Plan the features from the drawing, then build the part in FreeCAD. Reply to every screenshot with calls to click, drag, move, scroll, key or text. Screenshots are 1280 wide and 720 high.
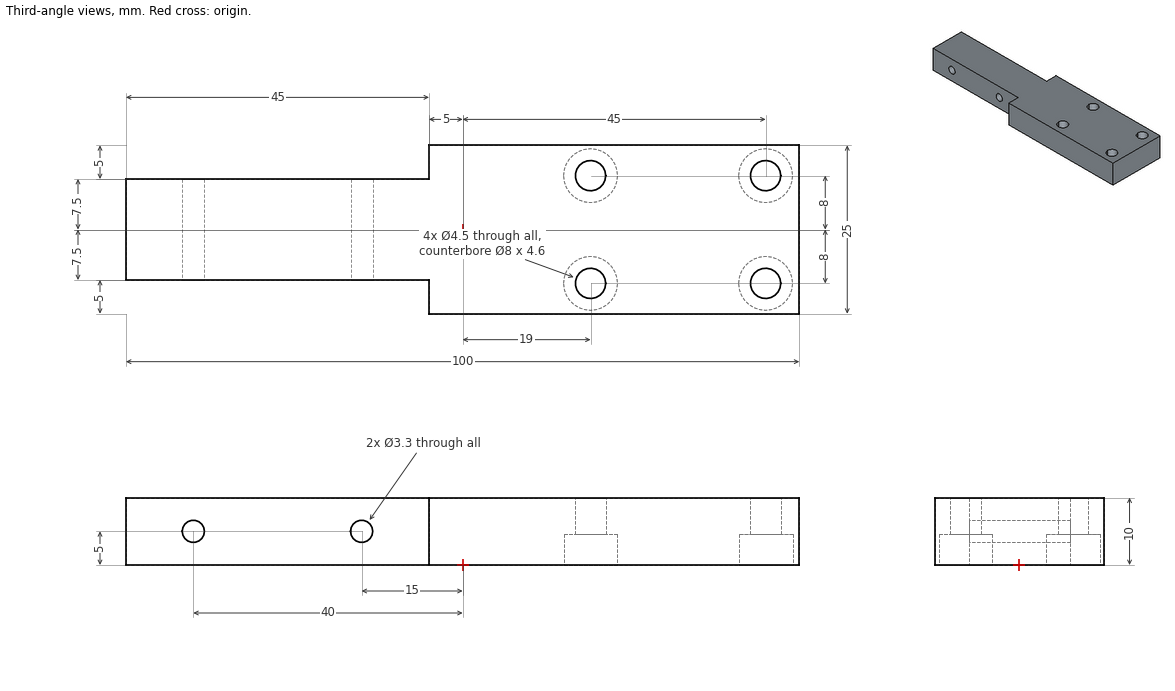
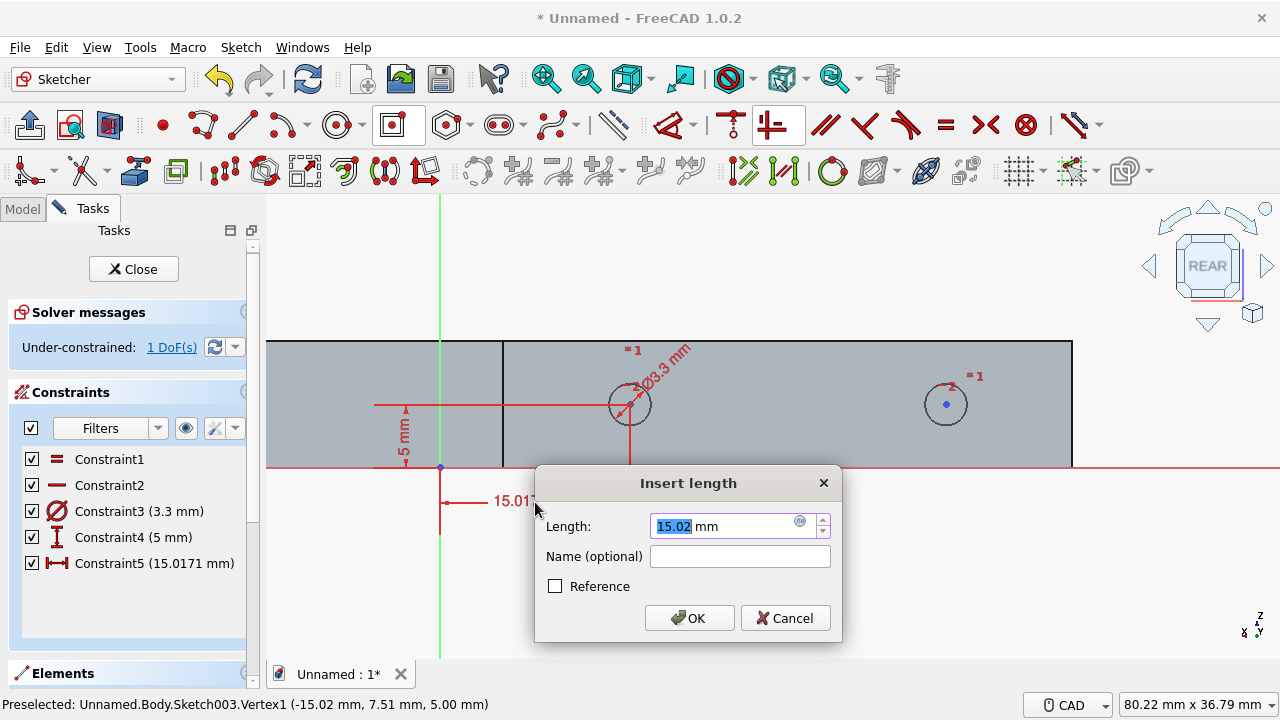
text(15)
key(Return)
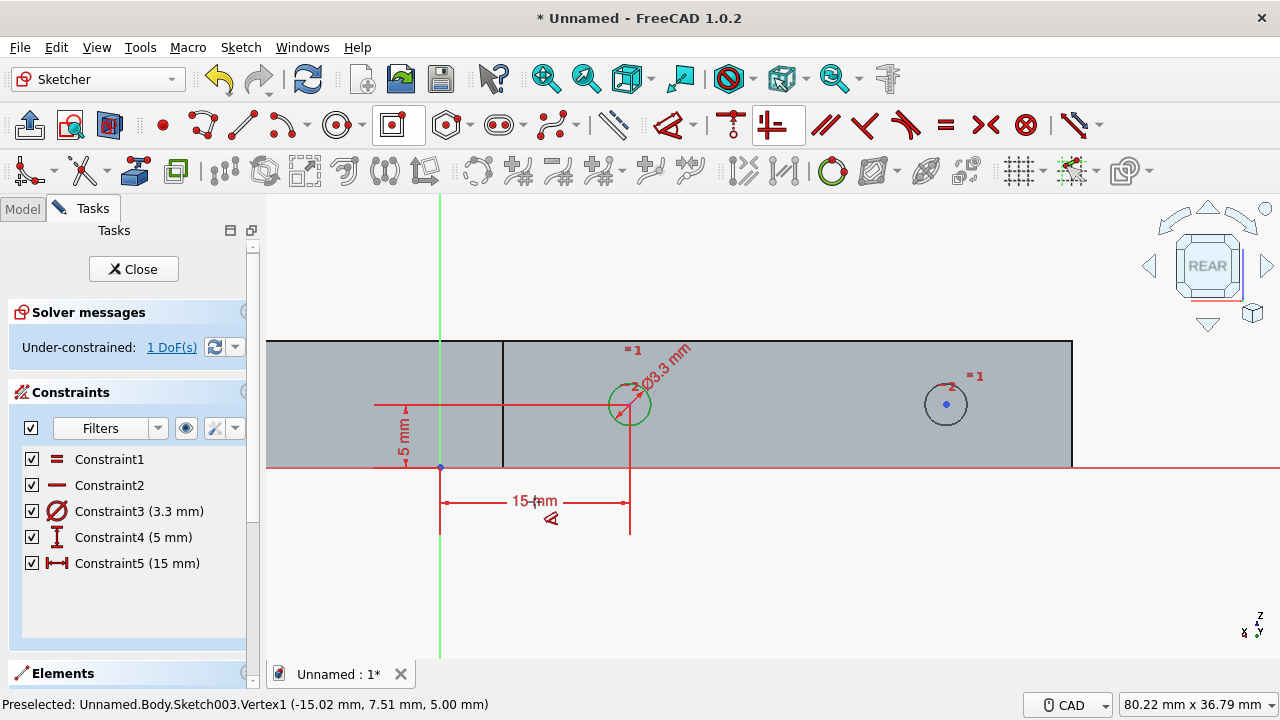
click(946, 405)
click(693, 502)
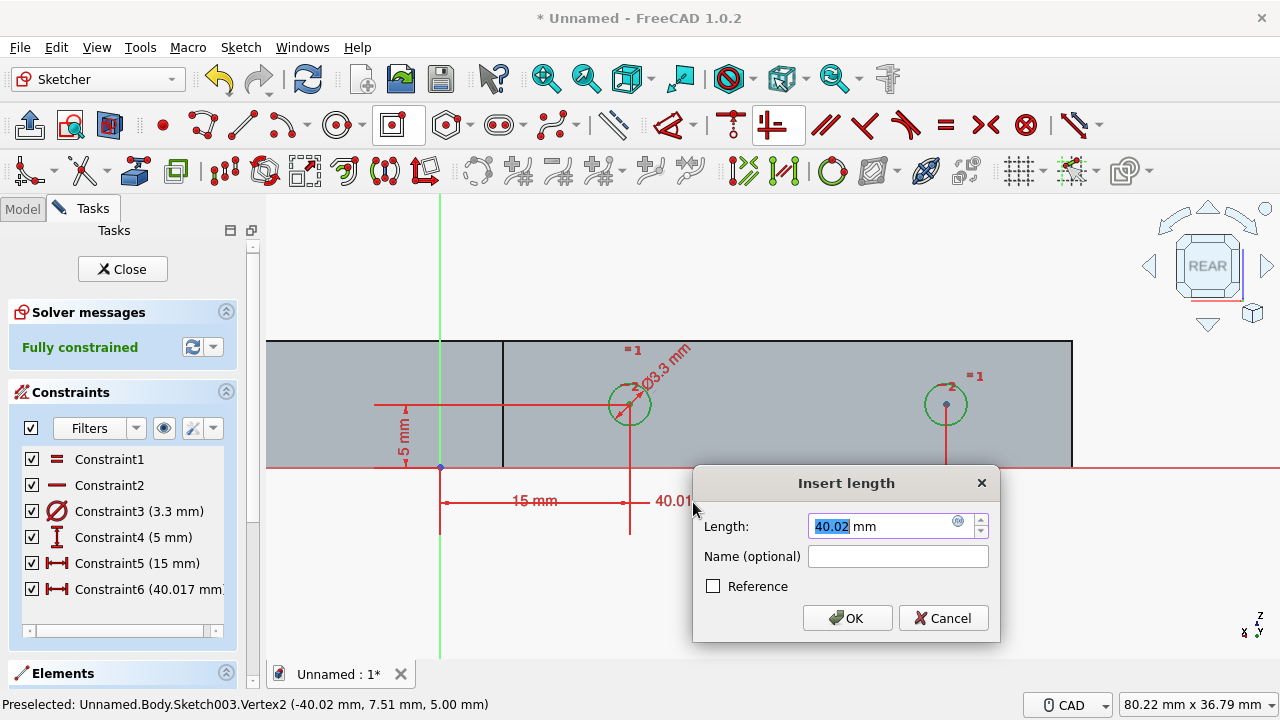
text(40)
key(Return)
key(Escape)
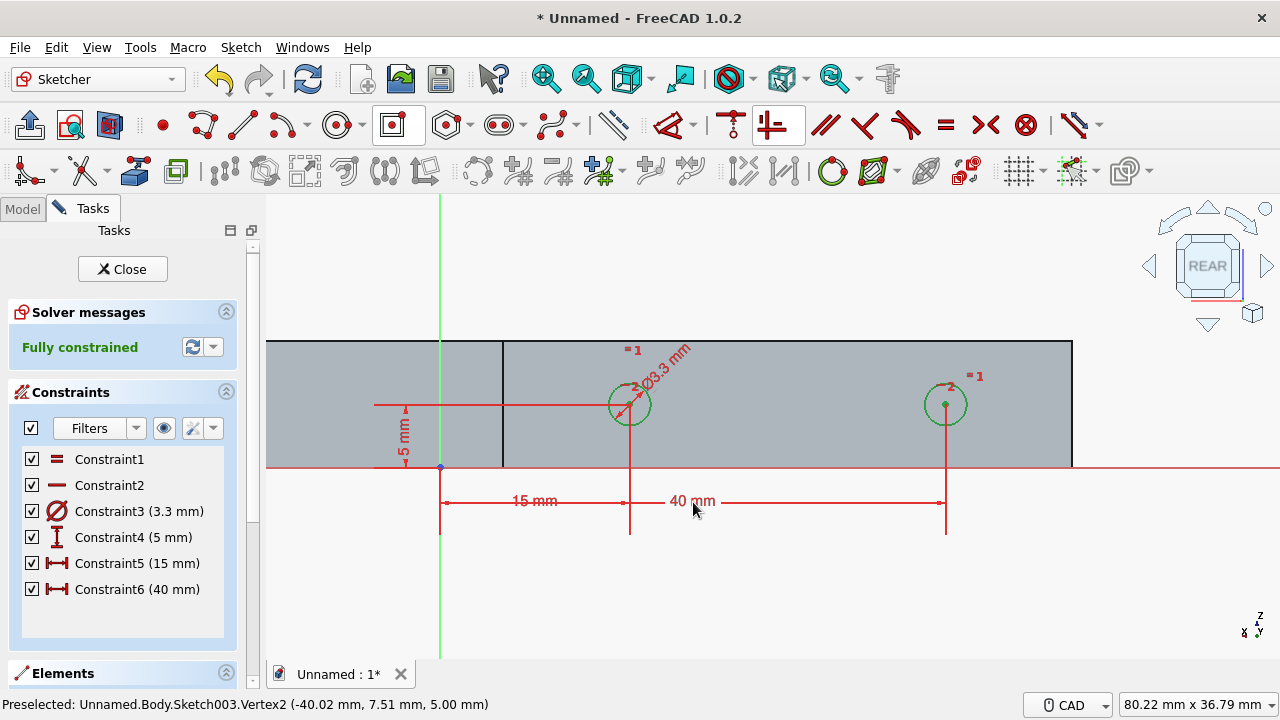
click(123, 269)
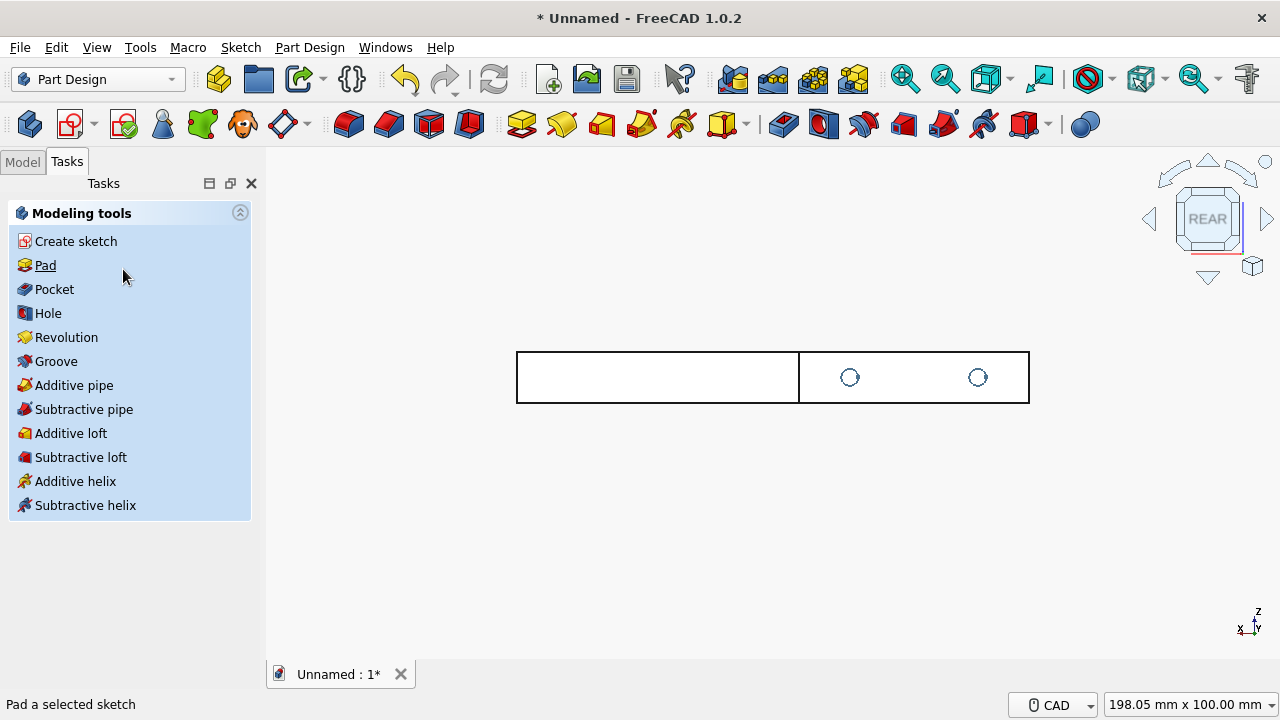
click(824, 124)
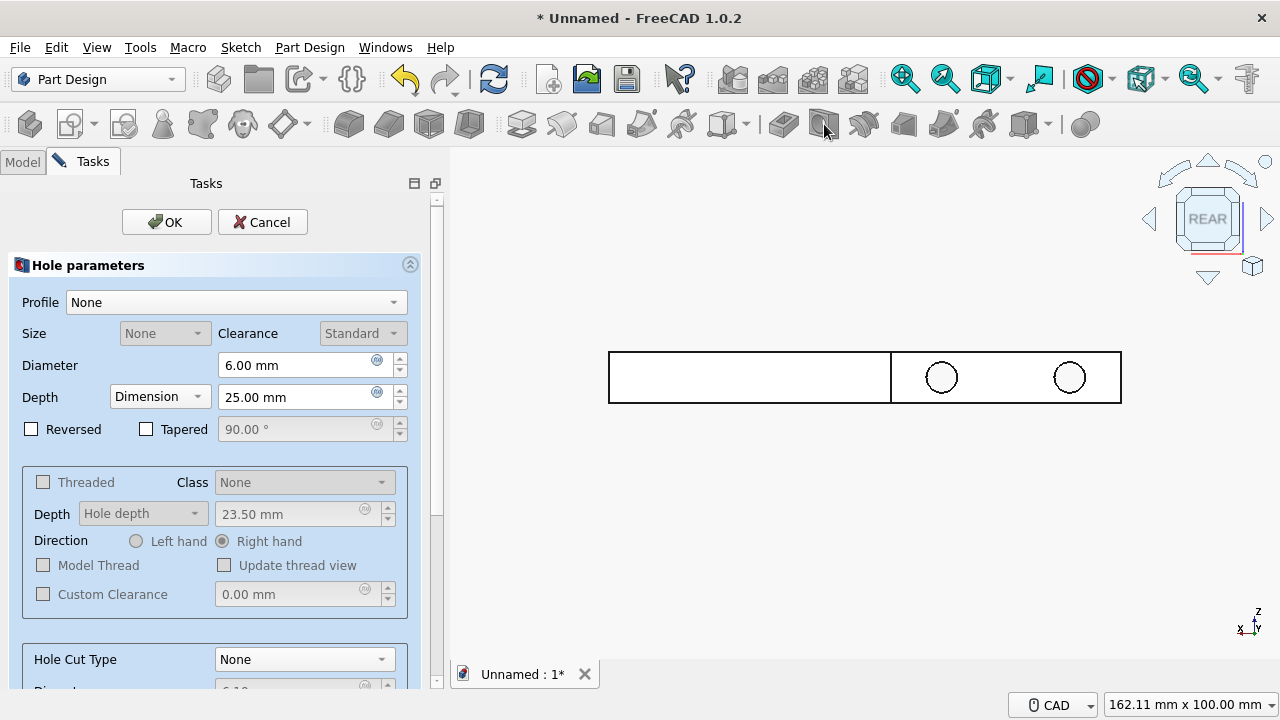
triple_click(305, 365)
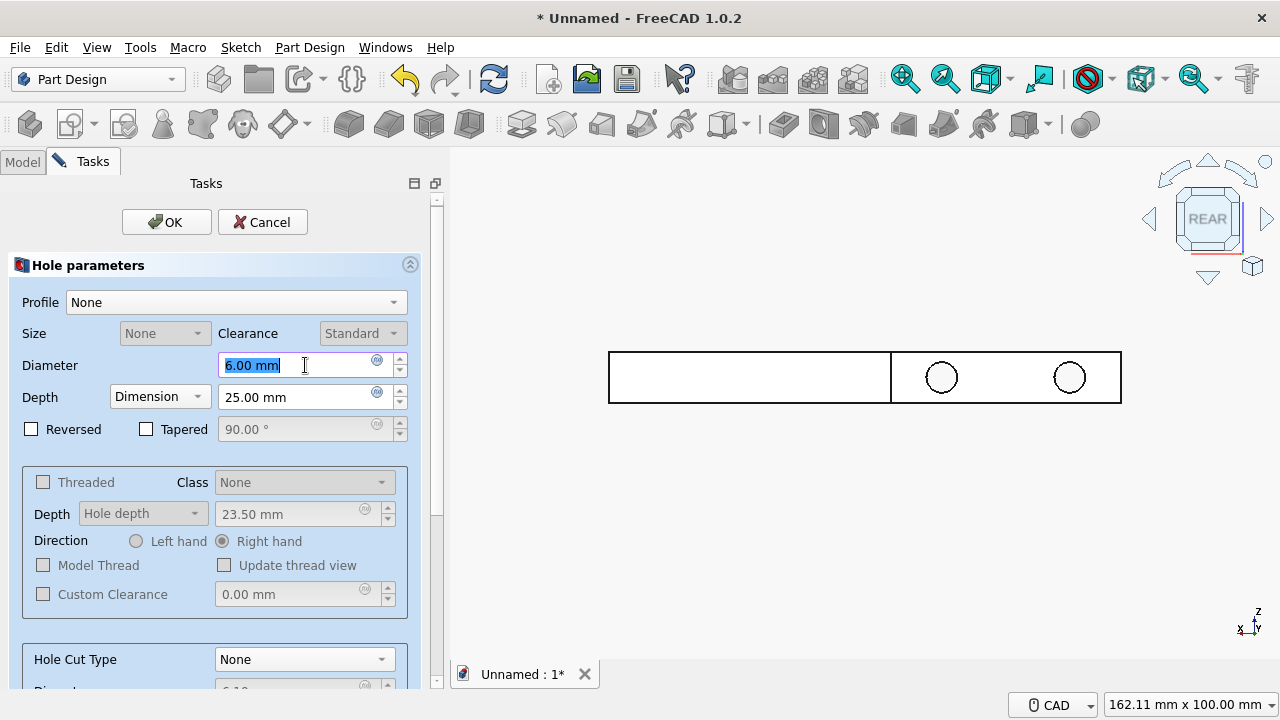
text(3.3)
key(Tab)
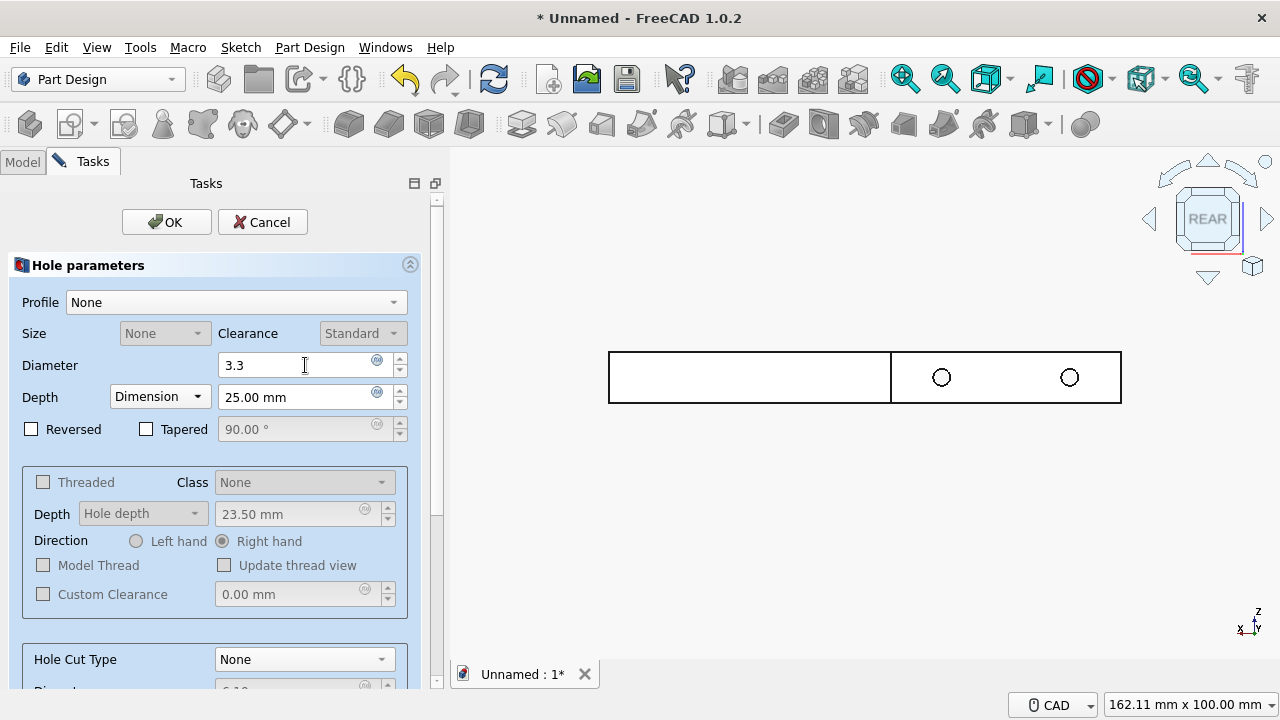
click(161, 396)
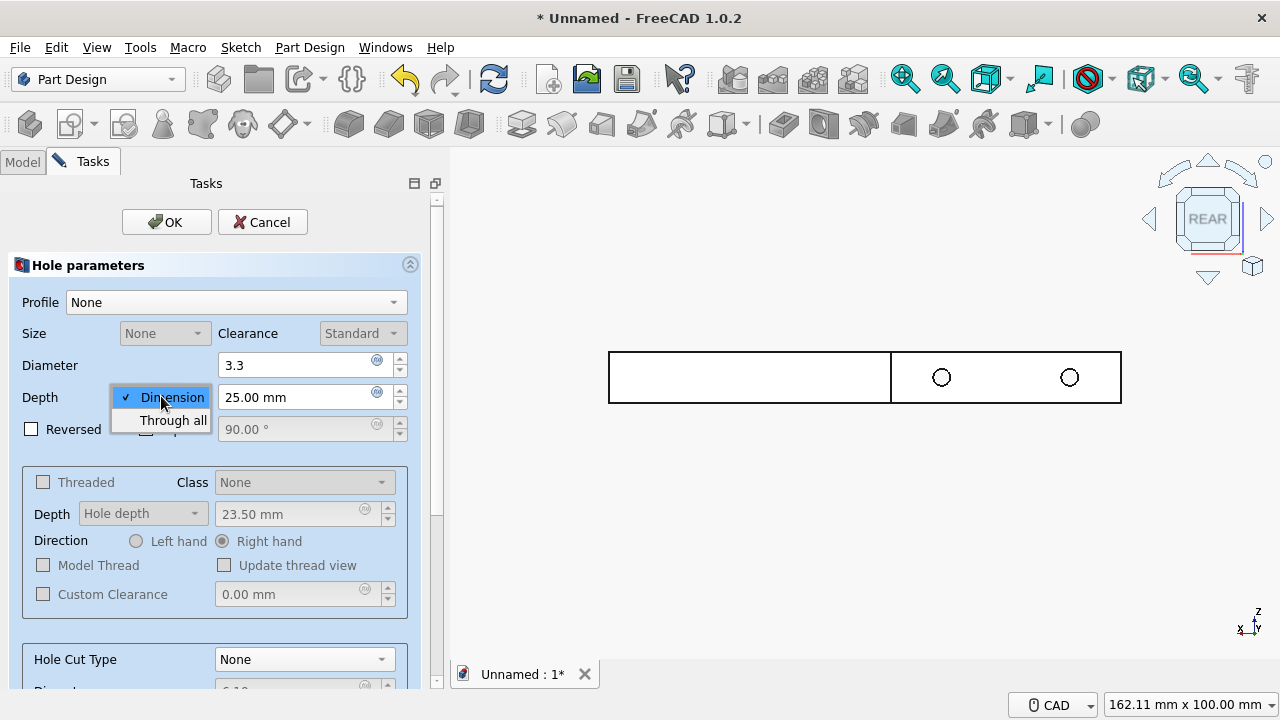
click(160, 420)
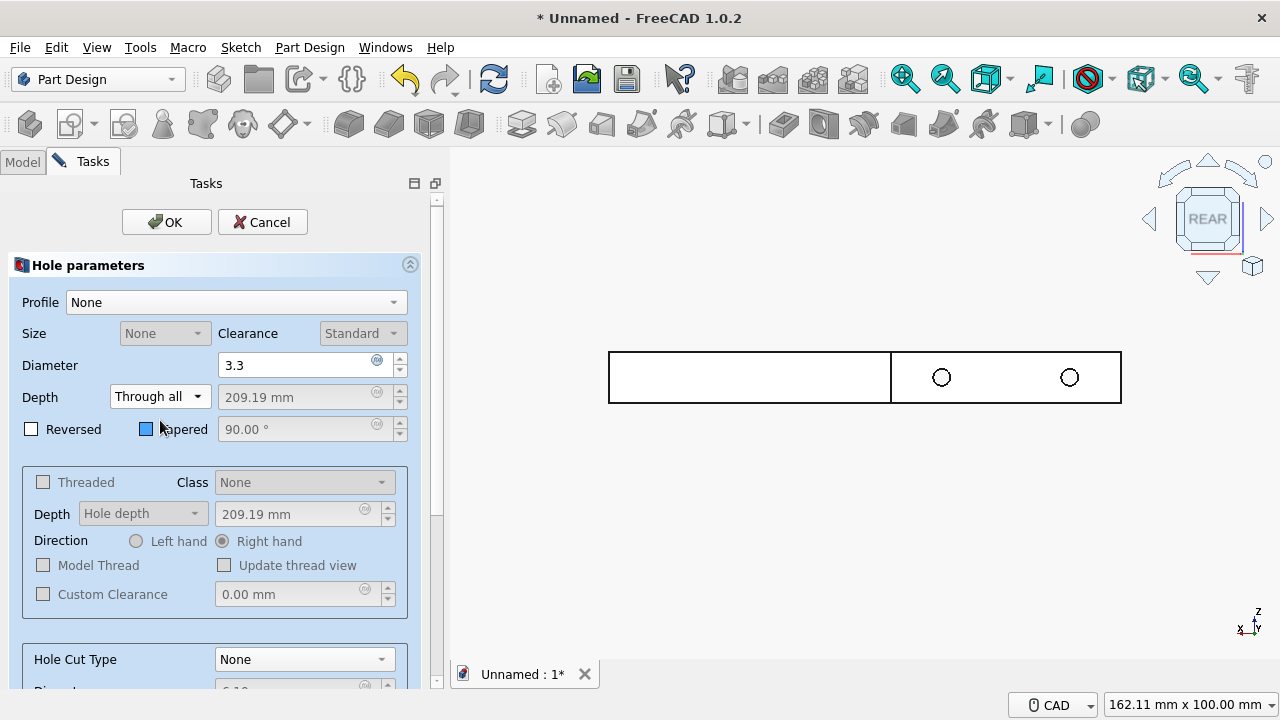
click(167, 222)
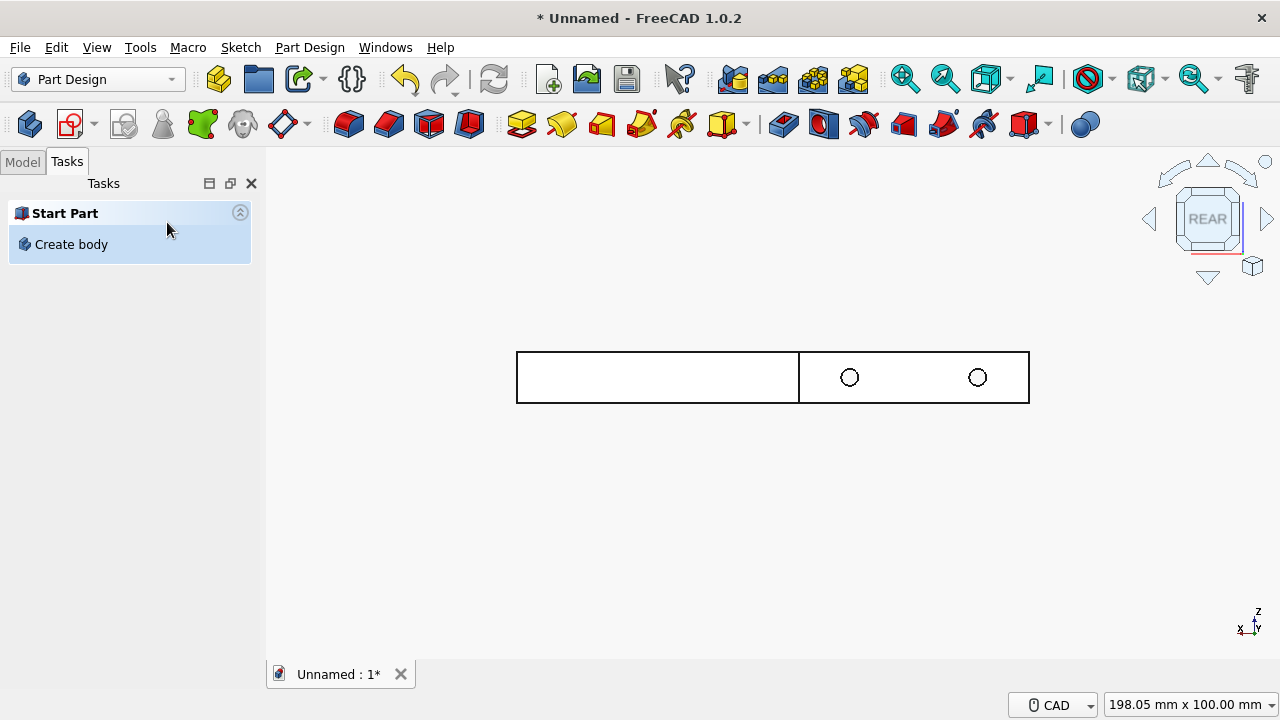
key(0)